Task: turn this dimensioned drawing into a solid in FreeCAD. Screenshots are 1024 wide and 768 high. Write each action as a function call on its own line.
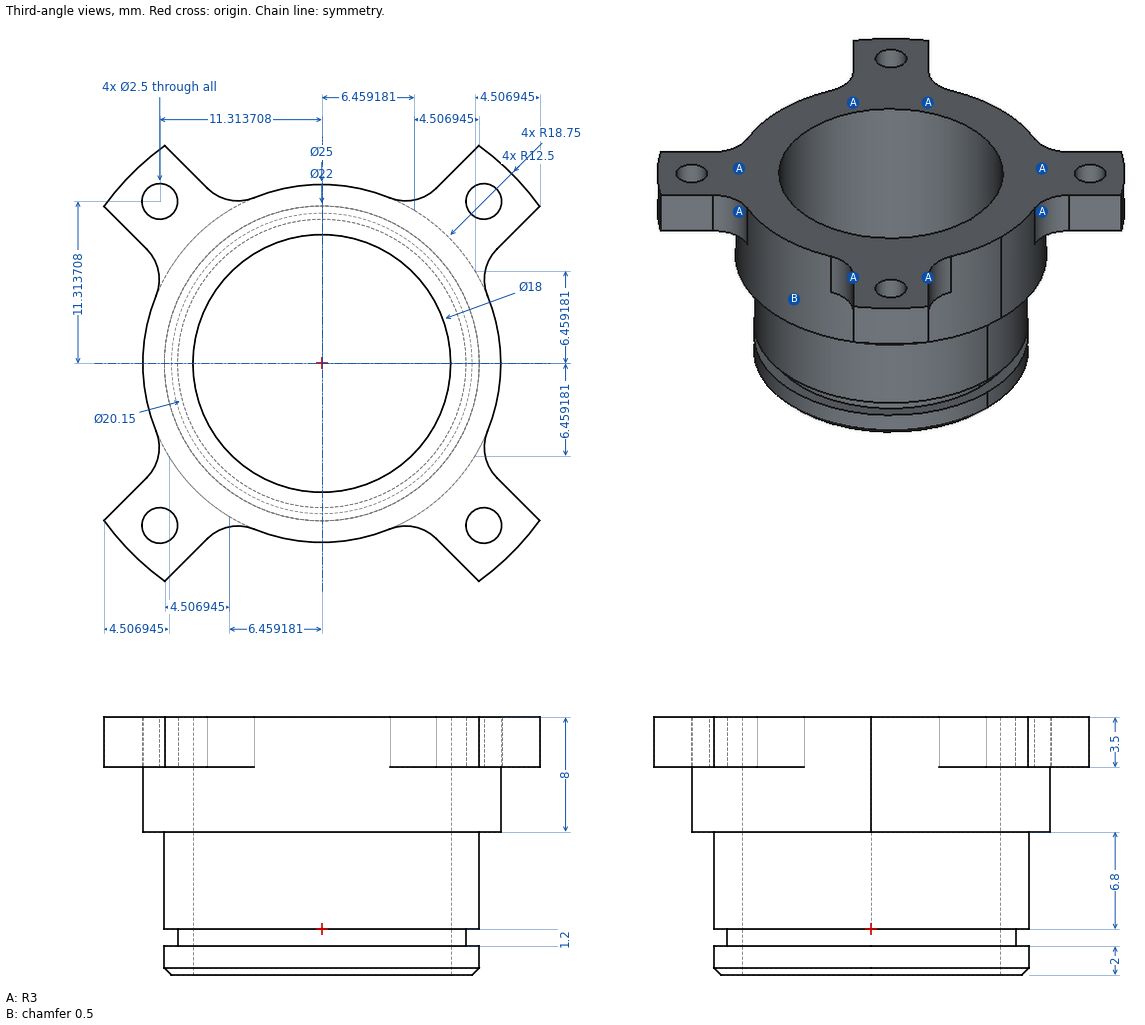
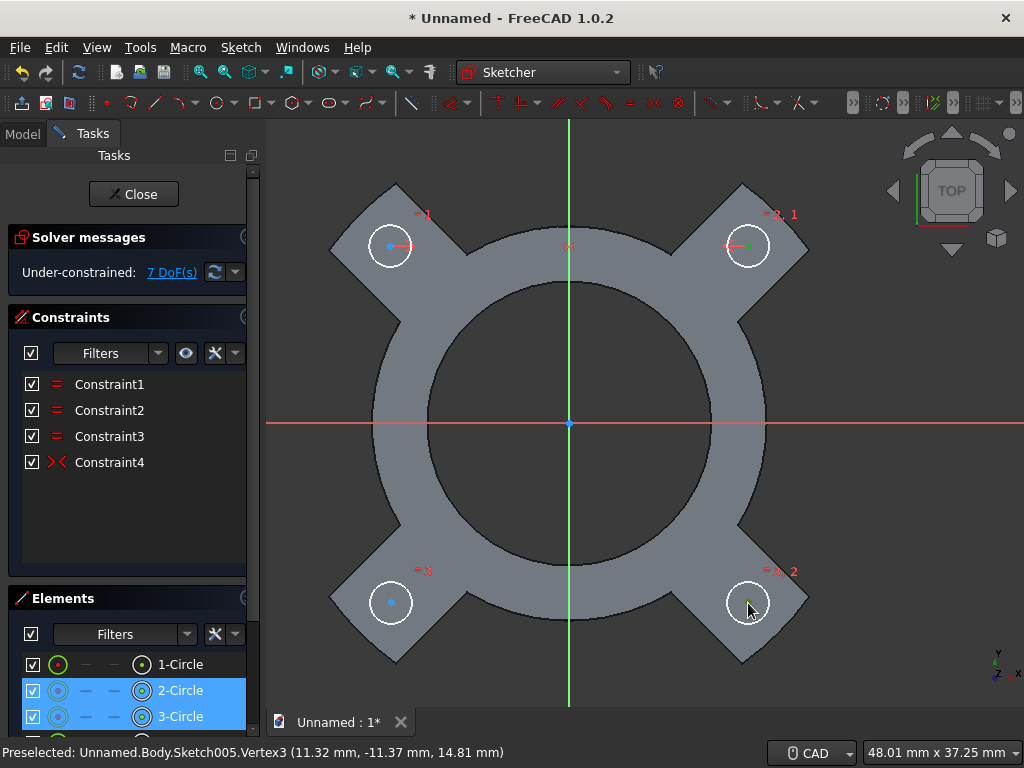
click(334, 423)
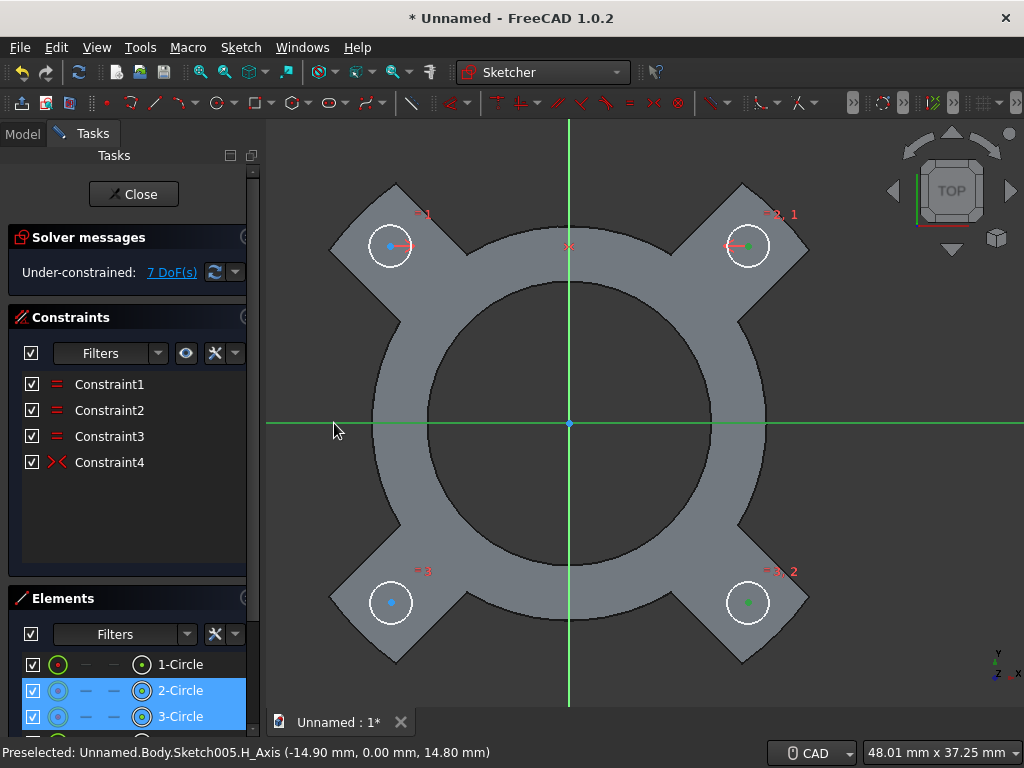
click(654, 104)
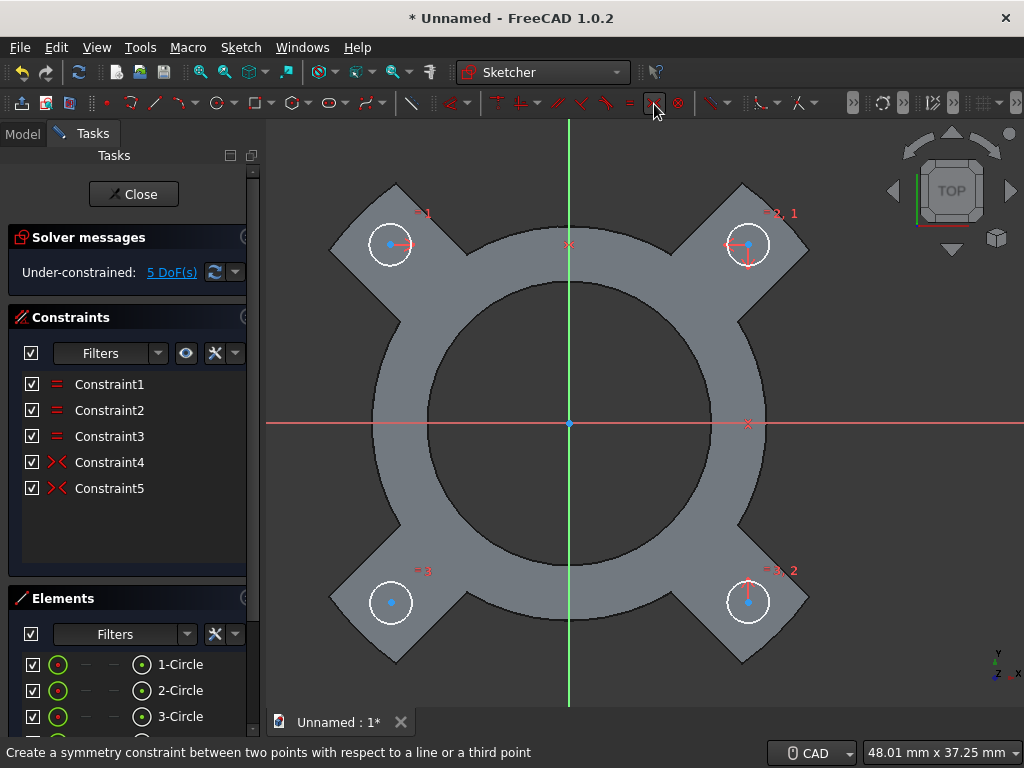
click(390, 245)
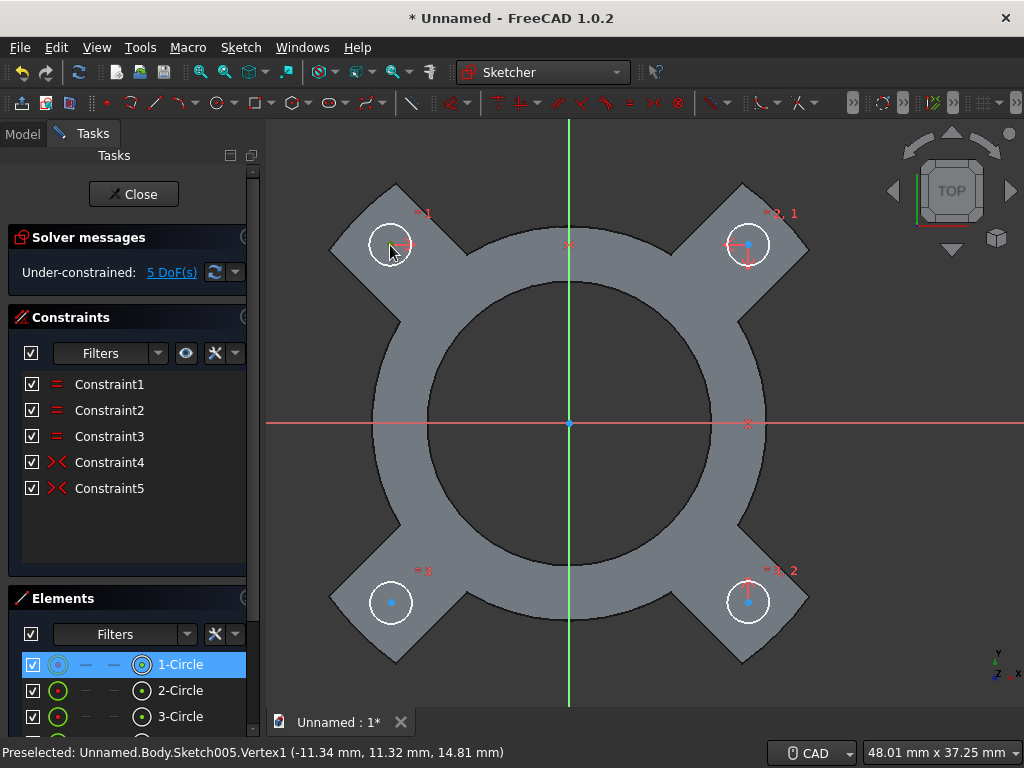
click(391, 603)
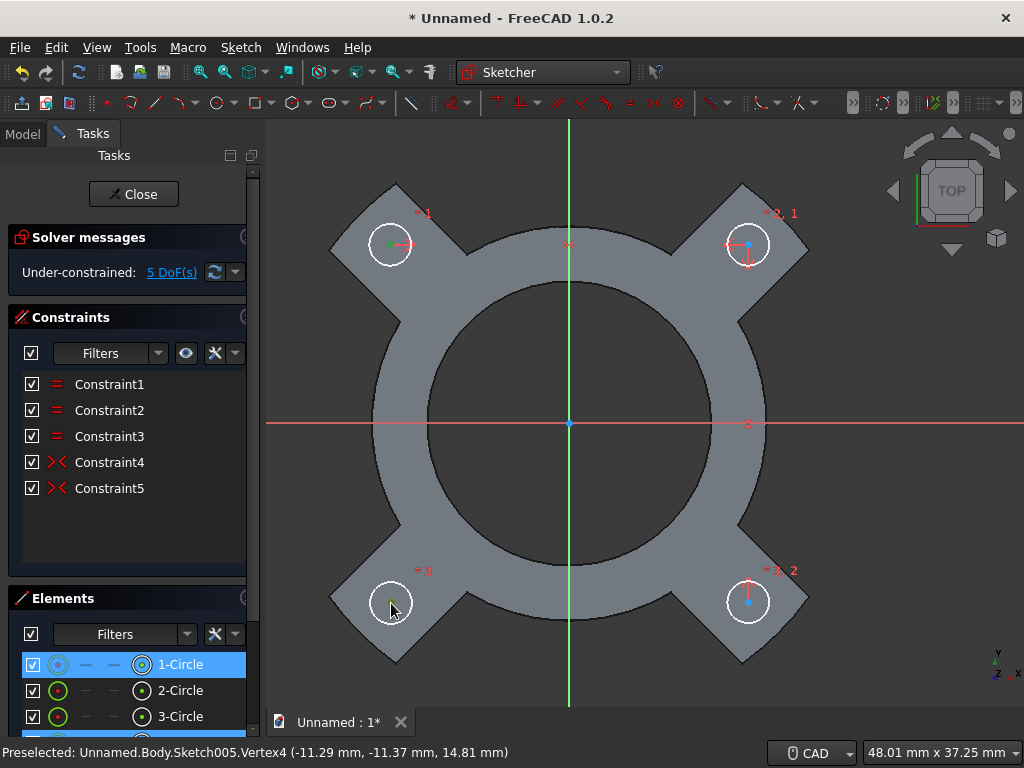
click(334, 423)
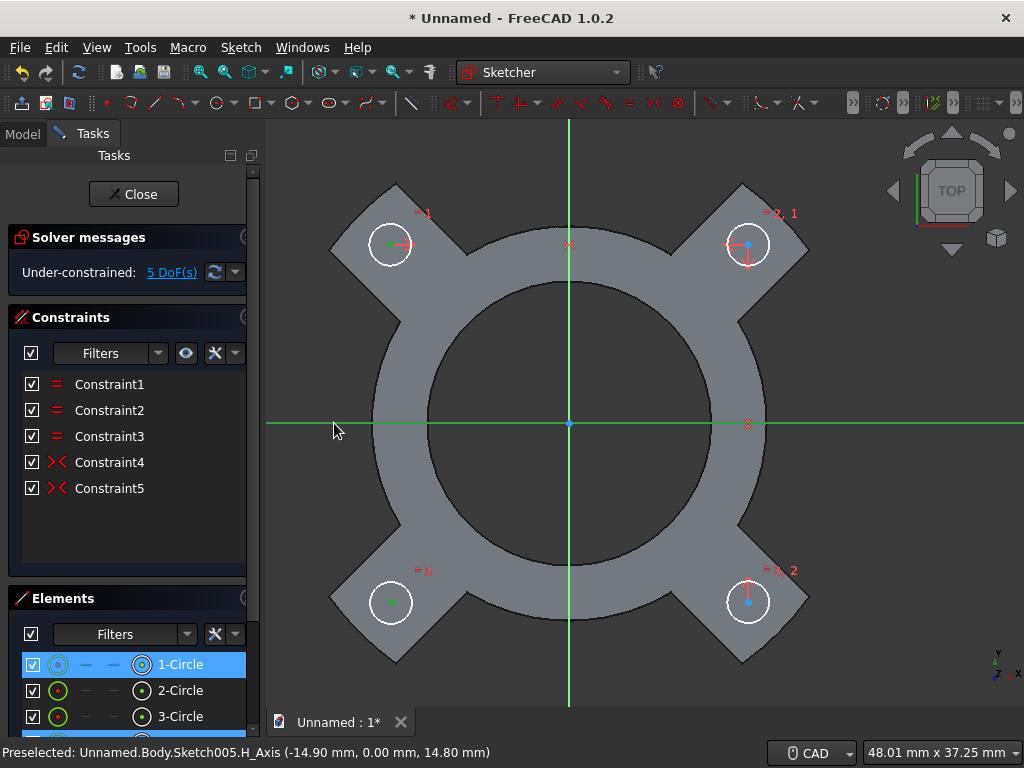
click(654, 104)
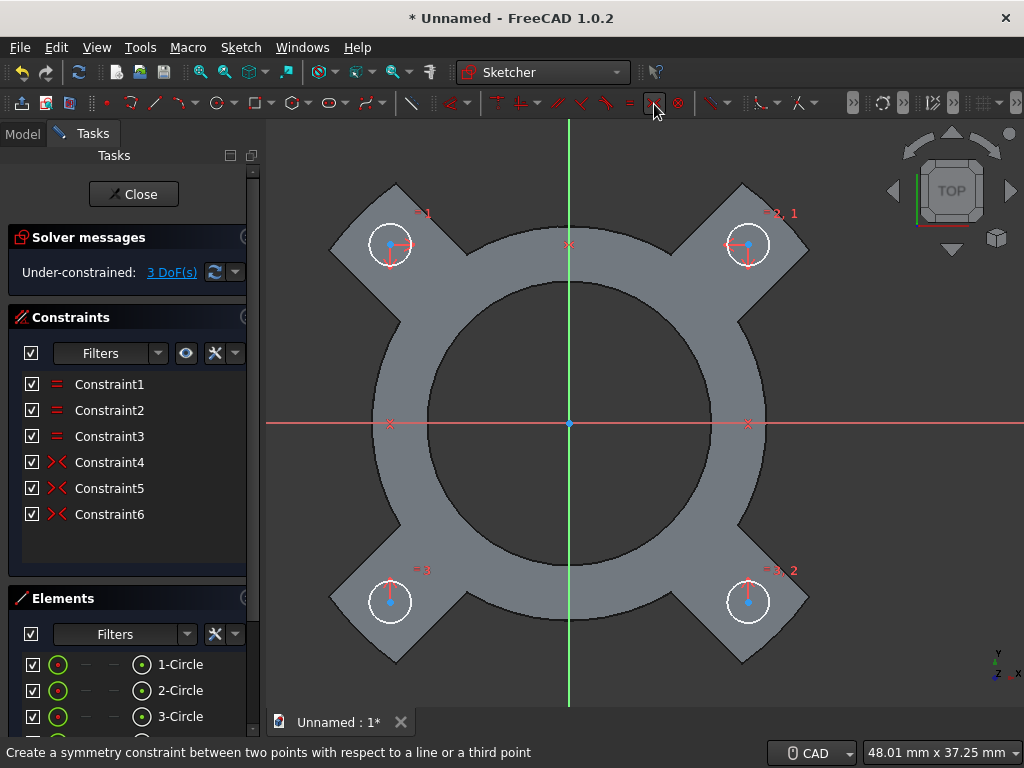
click(450, 104)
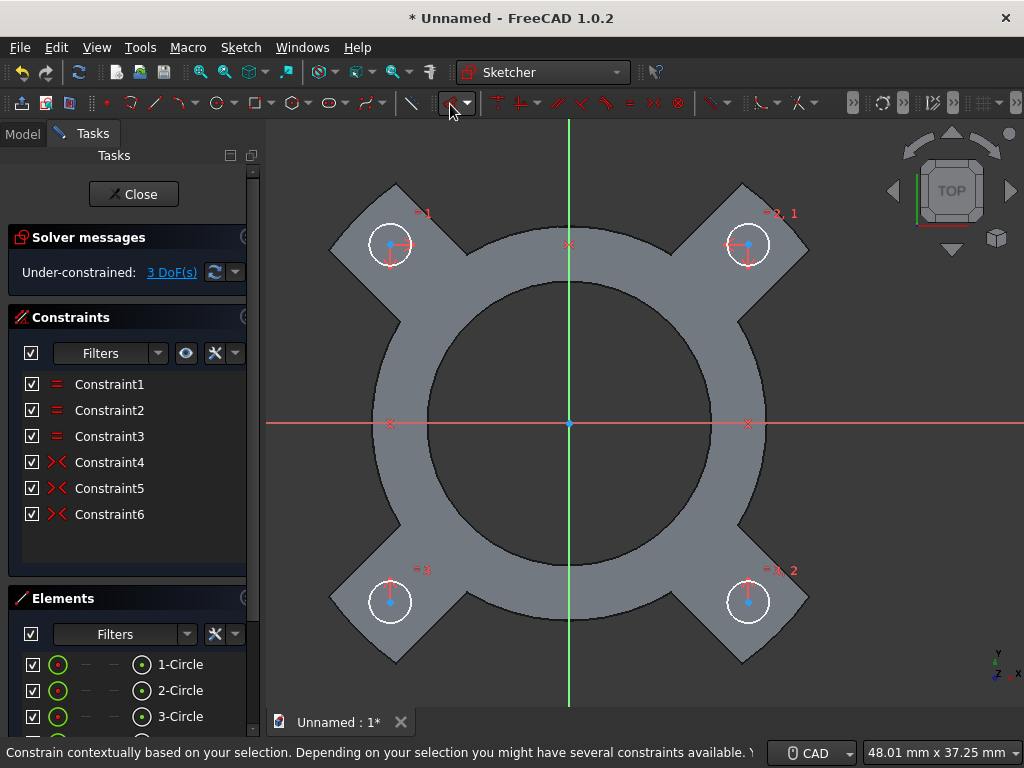
click(405, 230)
click(428, 207)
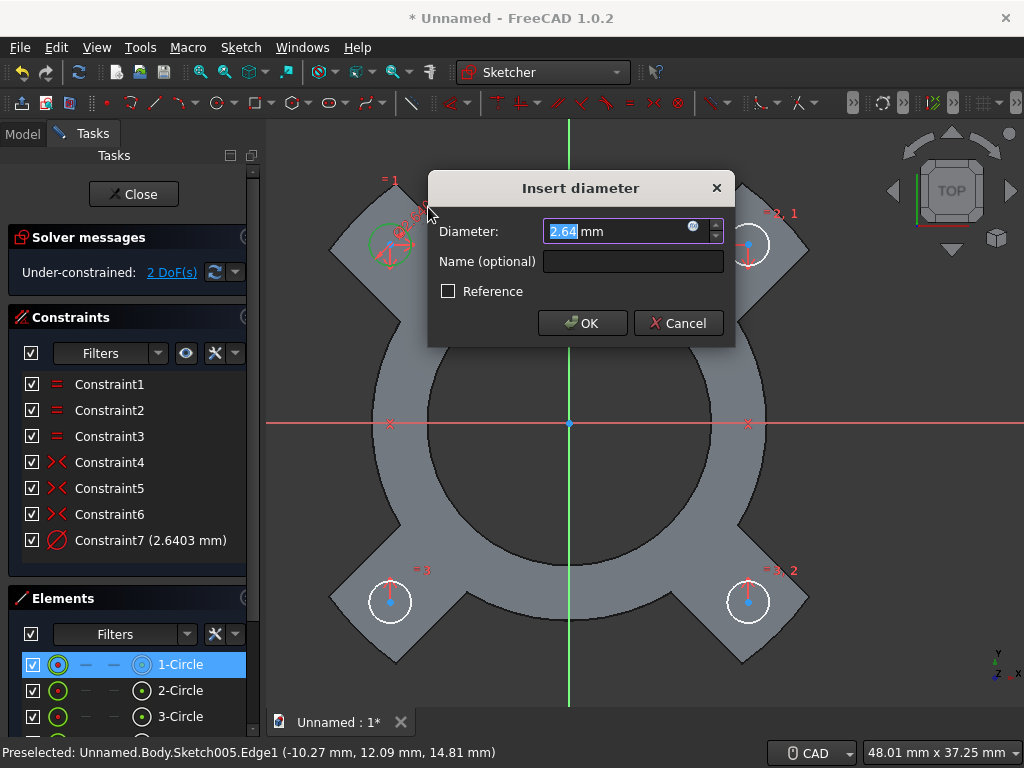
text(2.5)
key(Return)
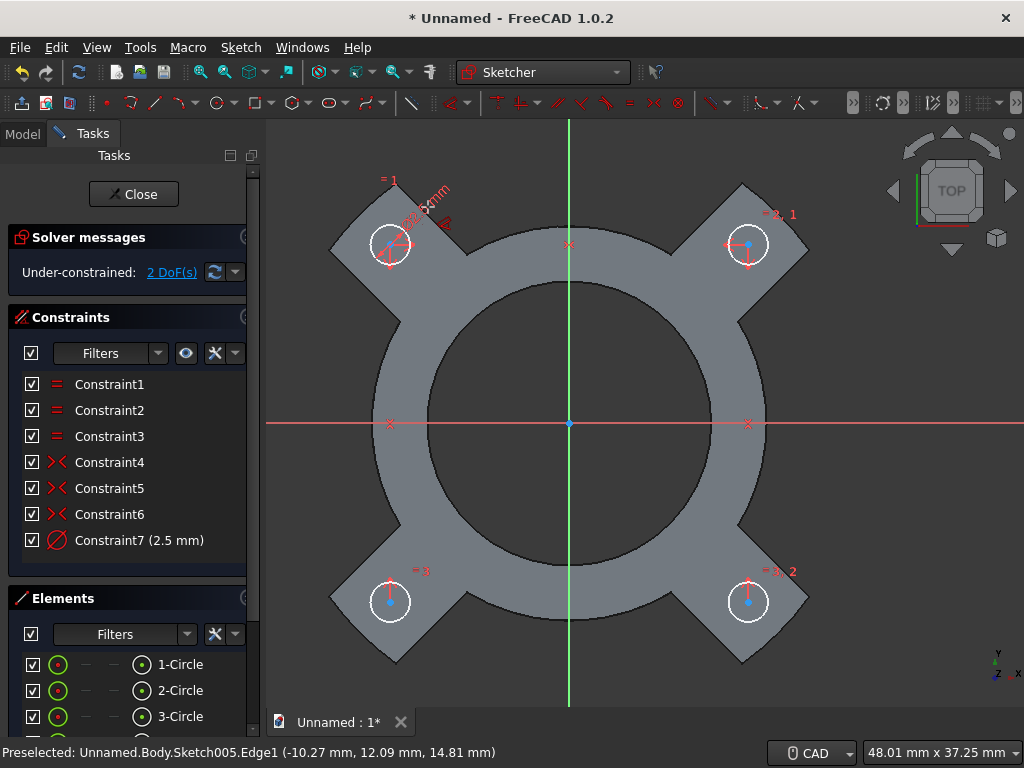
click(390, 245)
click(521, 211)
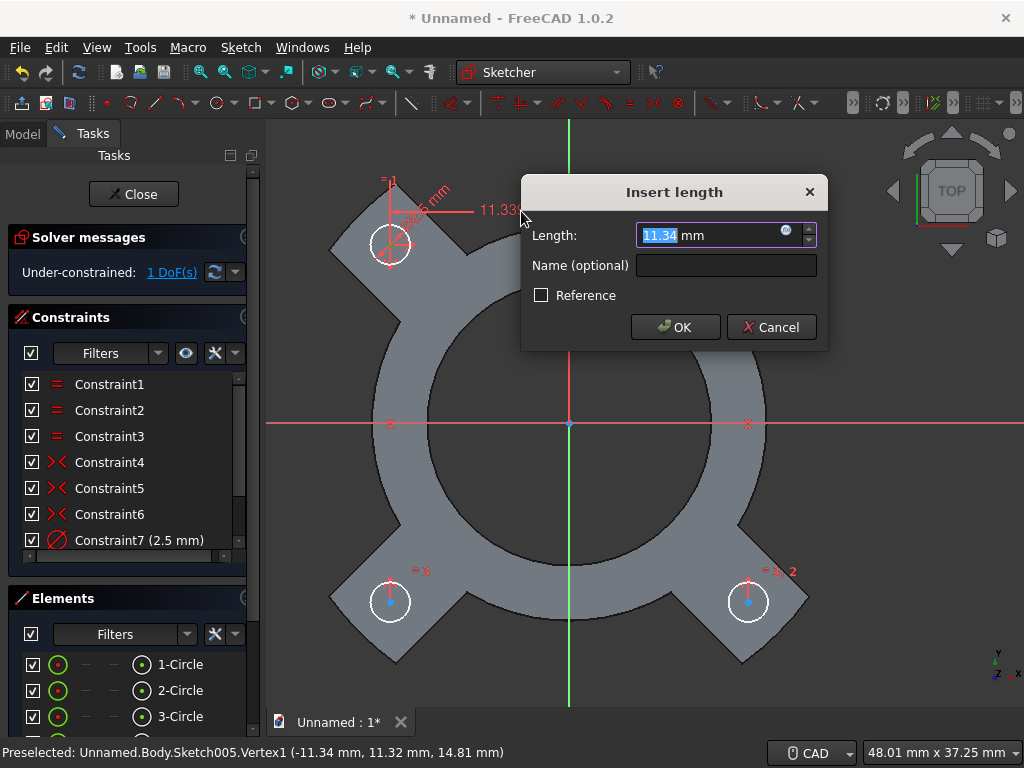
text(11.313708)
key(Return)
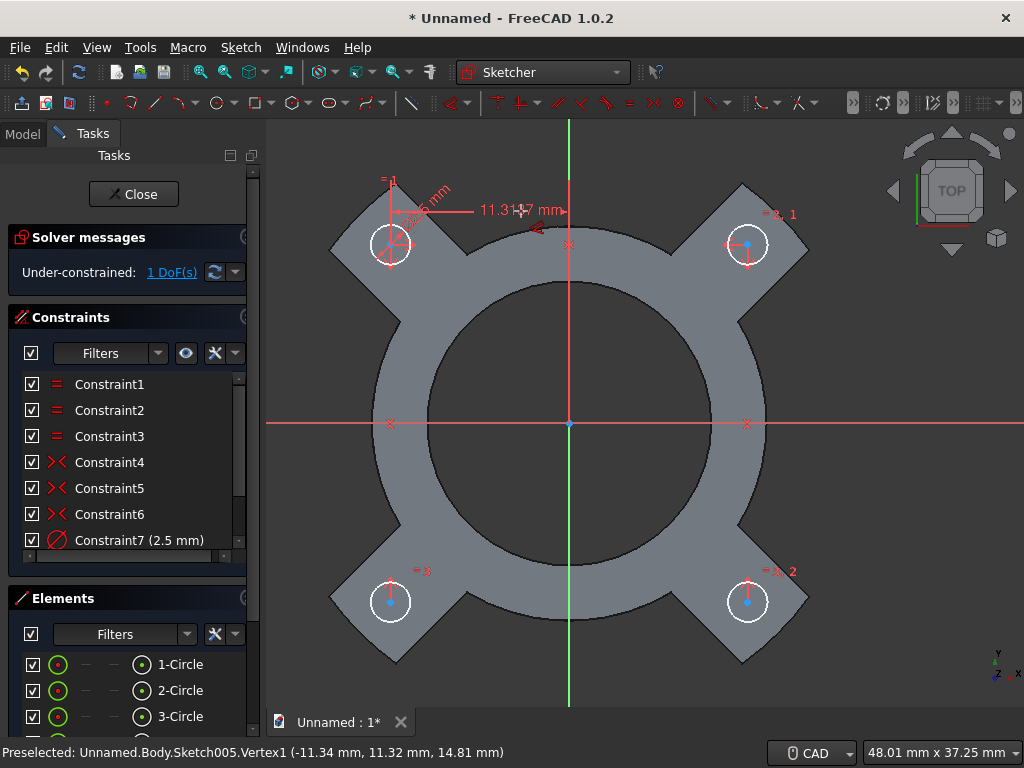
click(391, 245)
click(357, 334)